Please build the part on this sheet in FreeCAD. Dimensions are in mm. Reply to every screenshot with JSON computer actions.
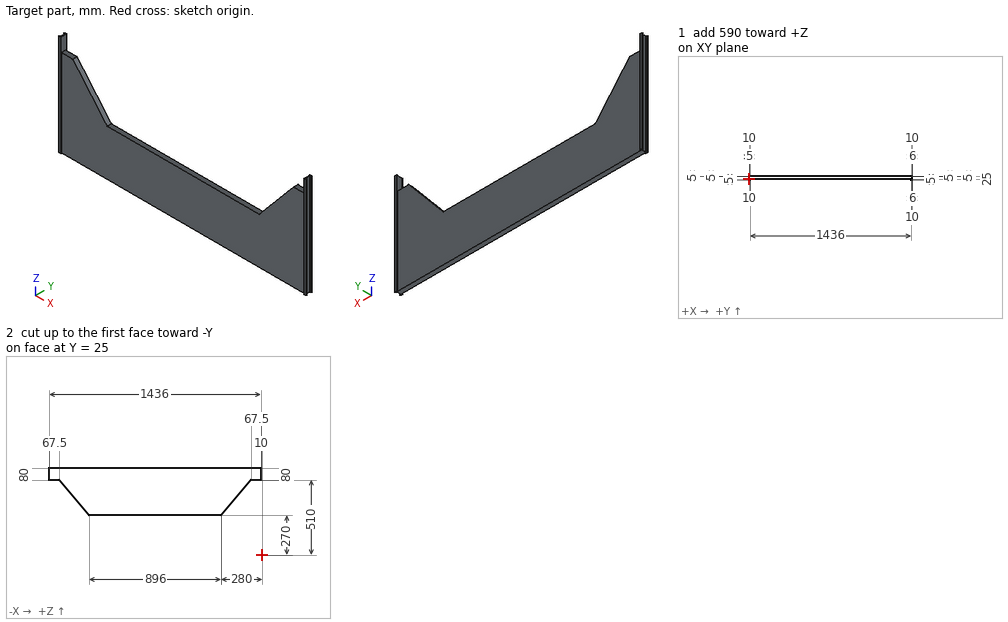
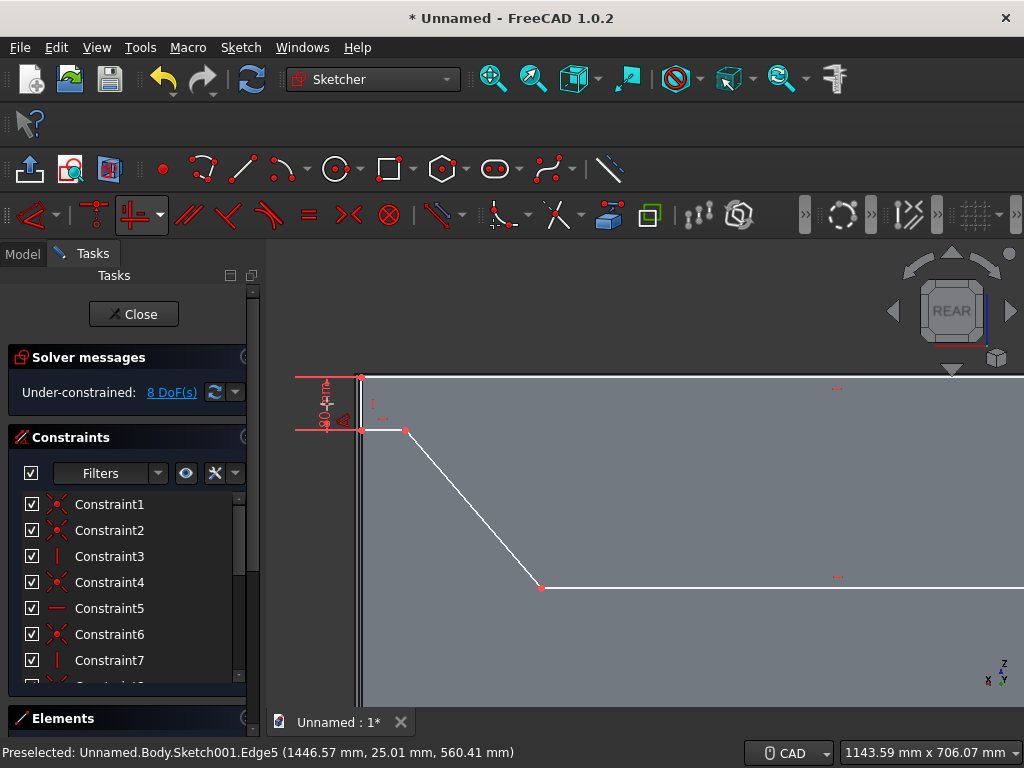
{"action": "left_click", "coordinate": [720, 588]}
{"action": "left_click", "coordinate": [700, 622]}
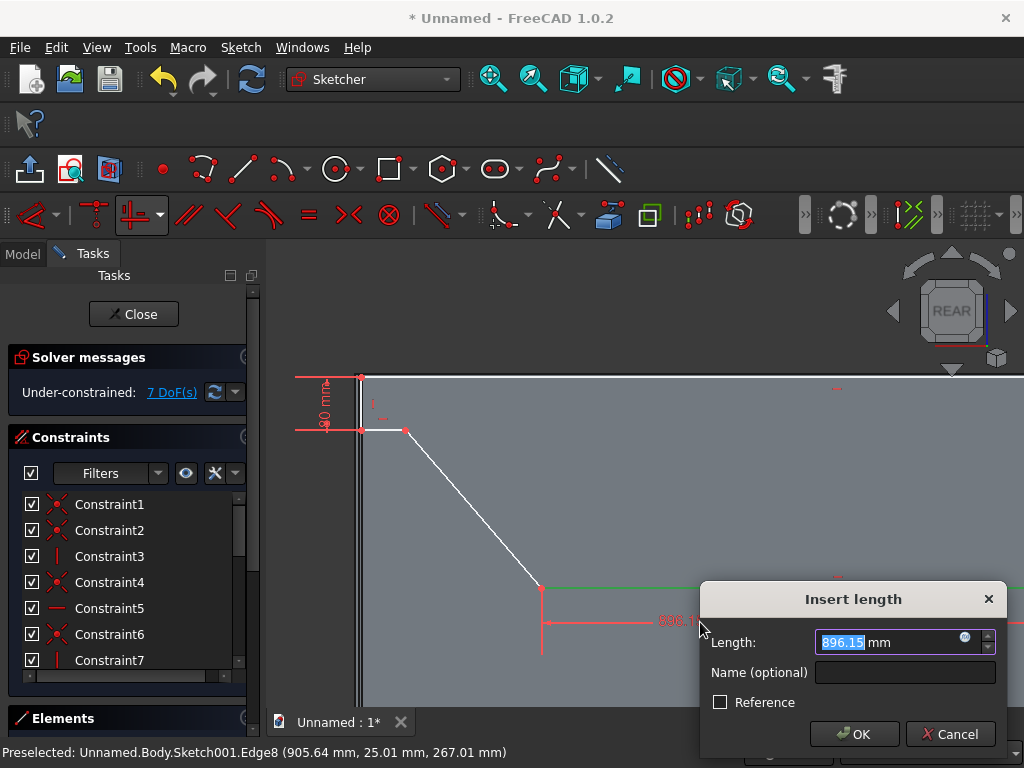
{"action": "type", "text": "896"}
{"action": "key", "text": "Return"}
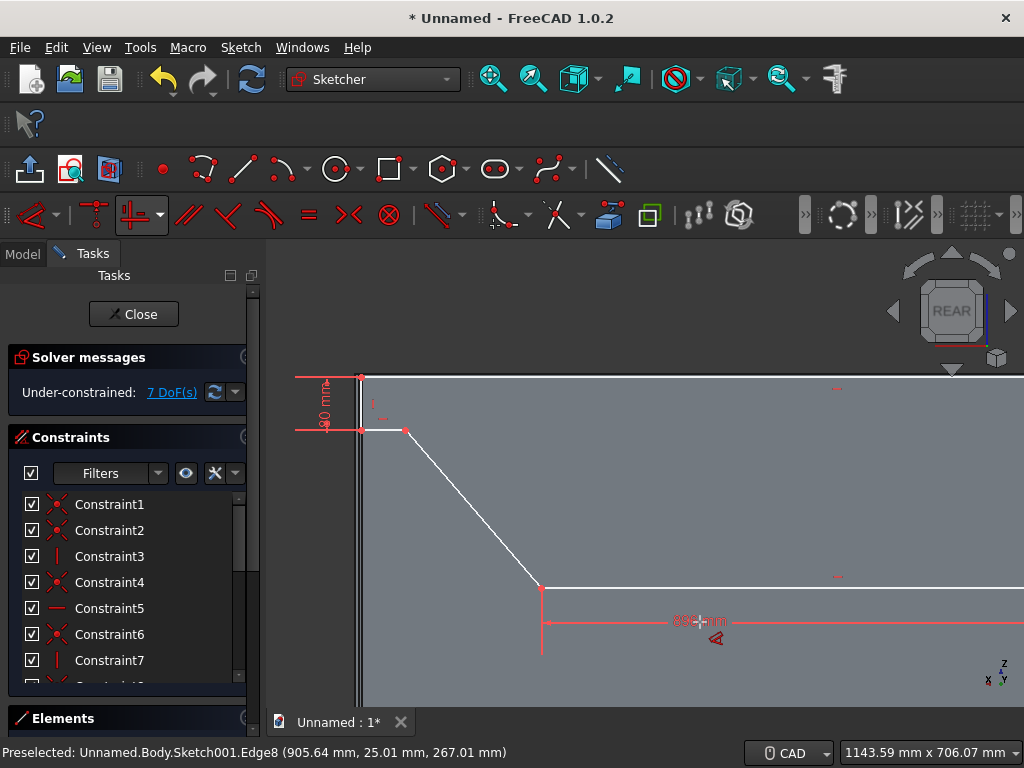
{"action": "scroll", "coordinate": [361, 394], "scroll_direction": "down", "scroll_amount": 4}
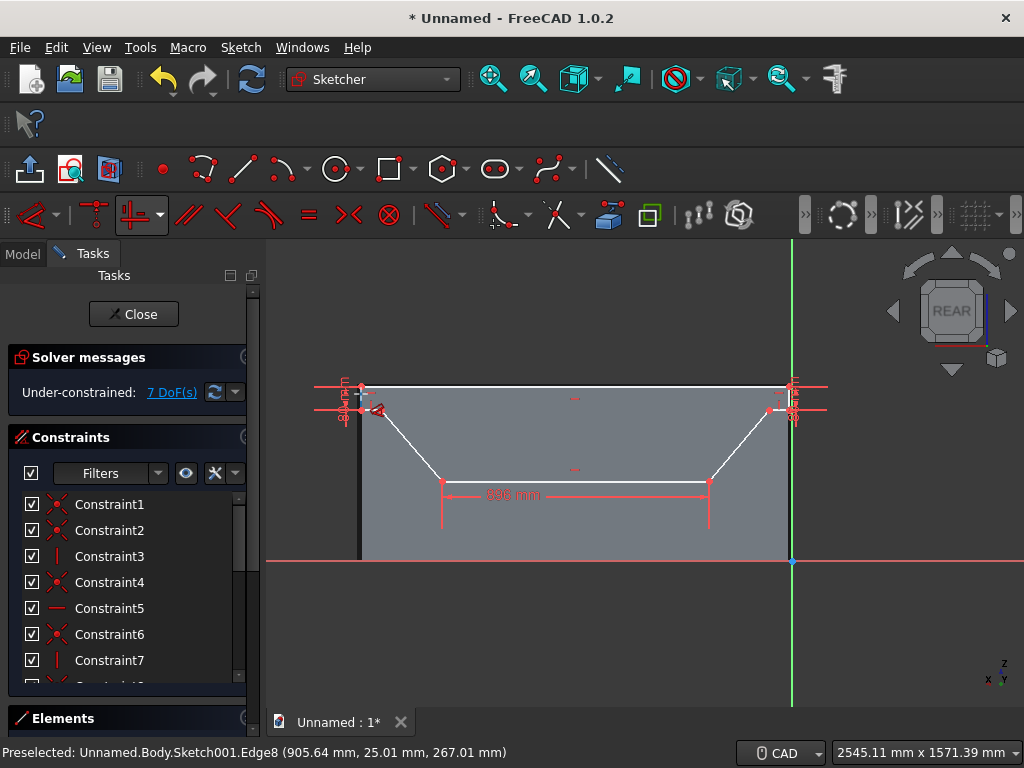
{"action": "scroll", "coordinate": [789, 410], "scroll_direction": "up", "scroll_amount": 13}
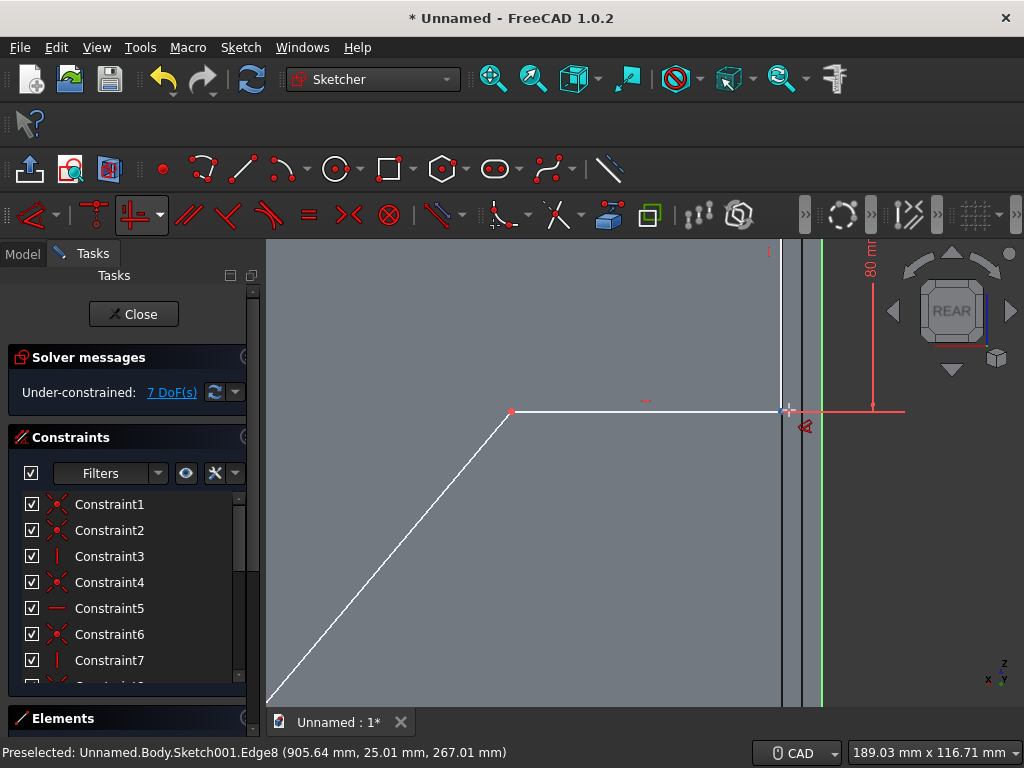
{"action": "left_click", "coordinate": [781, 412]}
{"action": "left_click", "coordinate": [802, 378]}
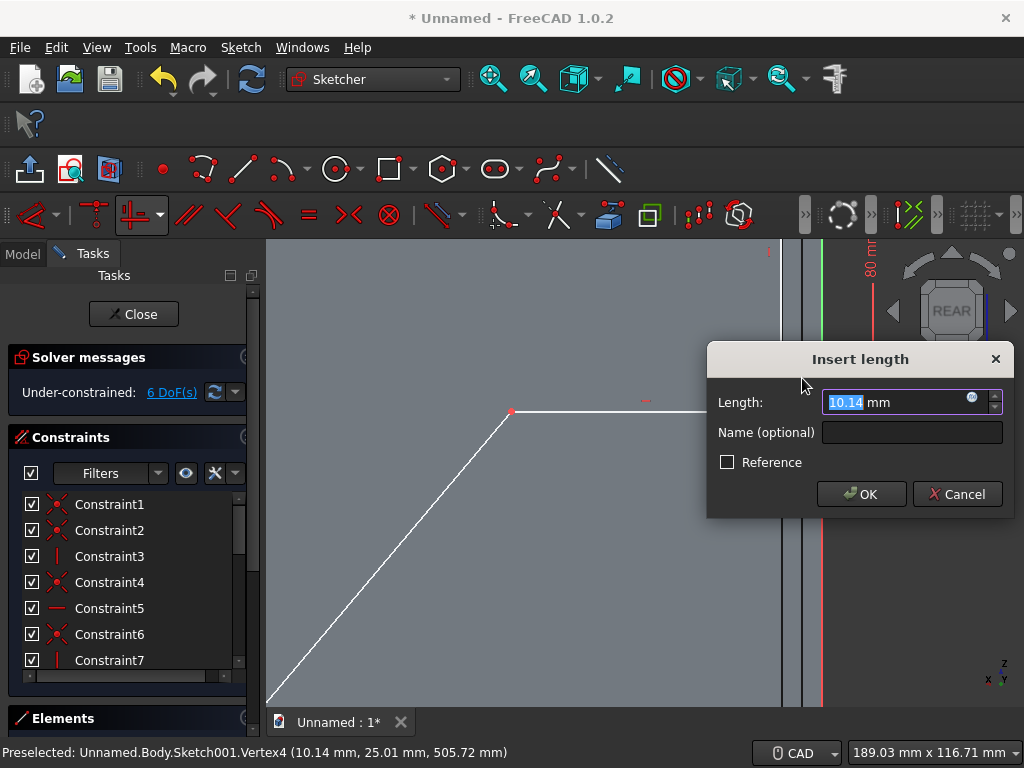
{"action": "type", "text": "10"}
{"action": "key", "text": "Return"}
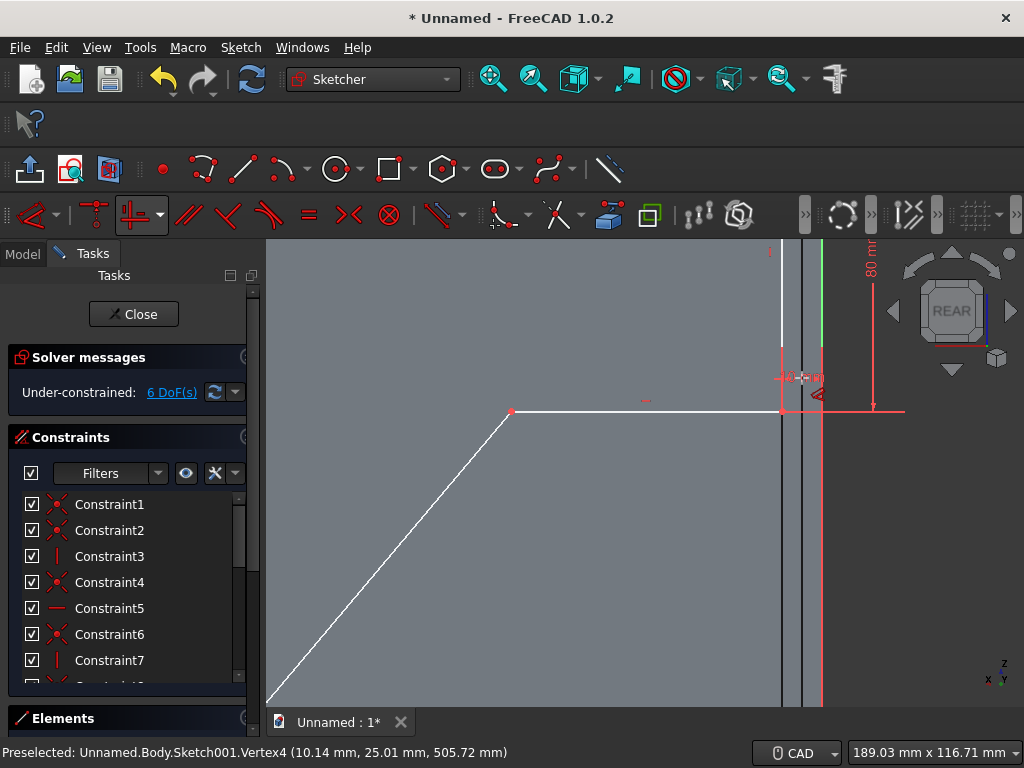
{"action": "scroll", "coordinate": [789, 410], "scroll_direction": "down", "scroll_amount": 13}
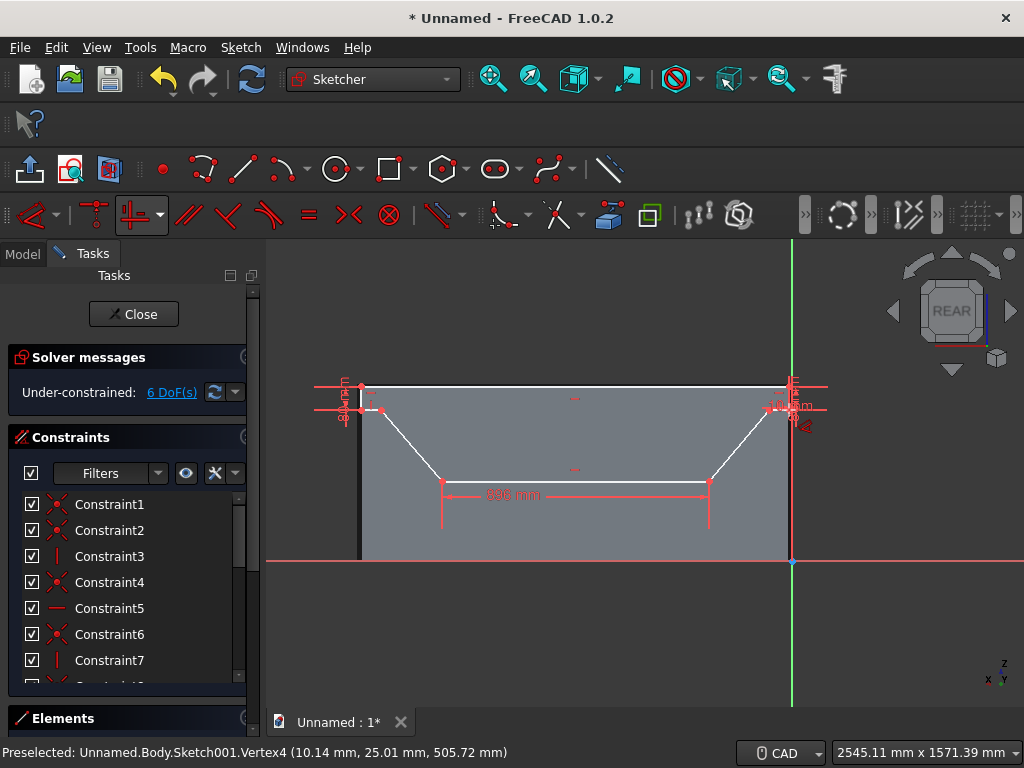
{"action": "scroll", "coordinate": [775, 410], "scroll_direction": "up", "scroll_amount": 5}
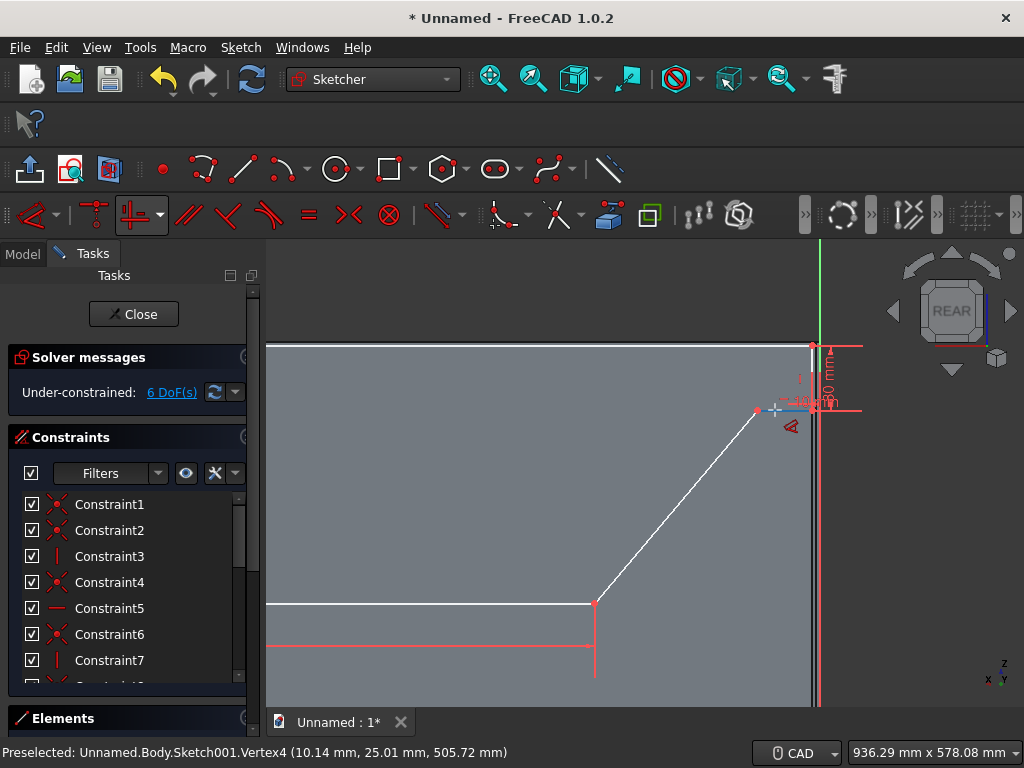
{"action": "left_click", "coordinate": [774, 411]}
{"action": "left_click", "coordinate": [785, 445]}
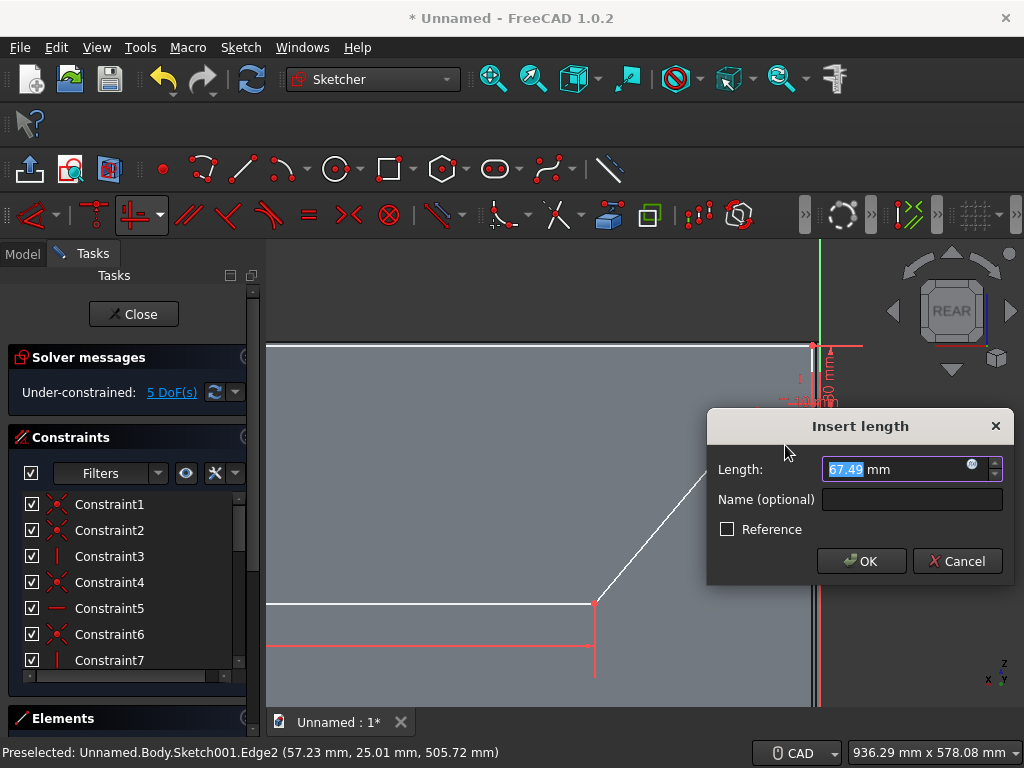
{"action": "type", "text": "67.5"}
{"action": "key", "text": "Return"}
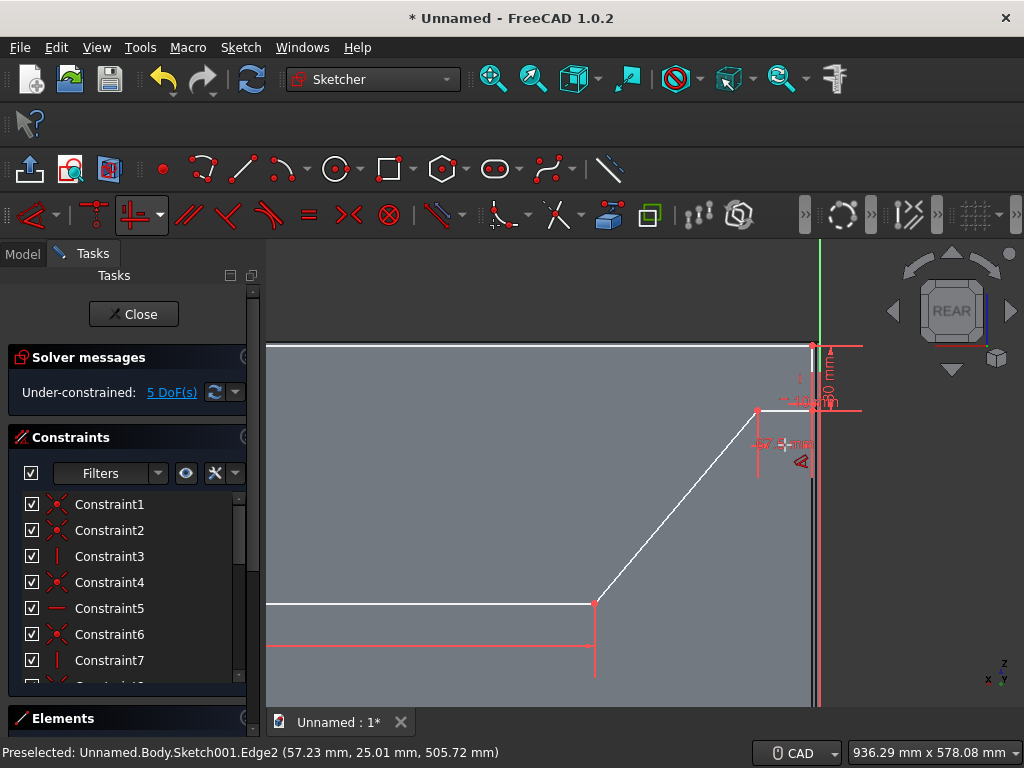
{"action": "left_click", "coordinate": [463, 346]}
{"action": "left_click", "coordinate": [553, 312]}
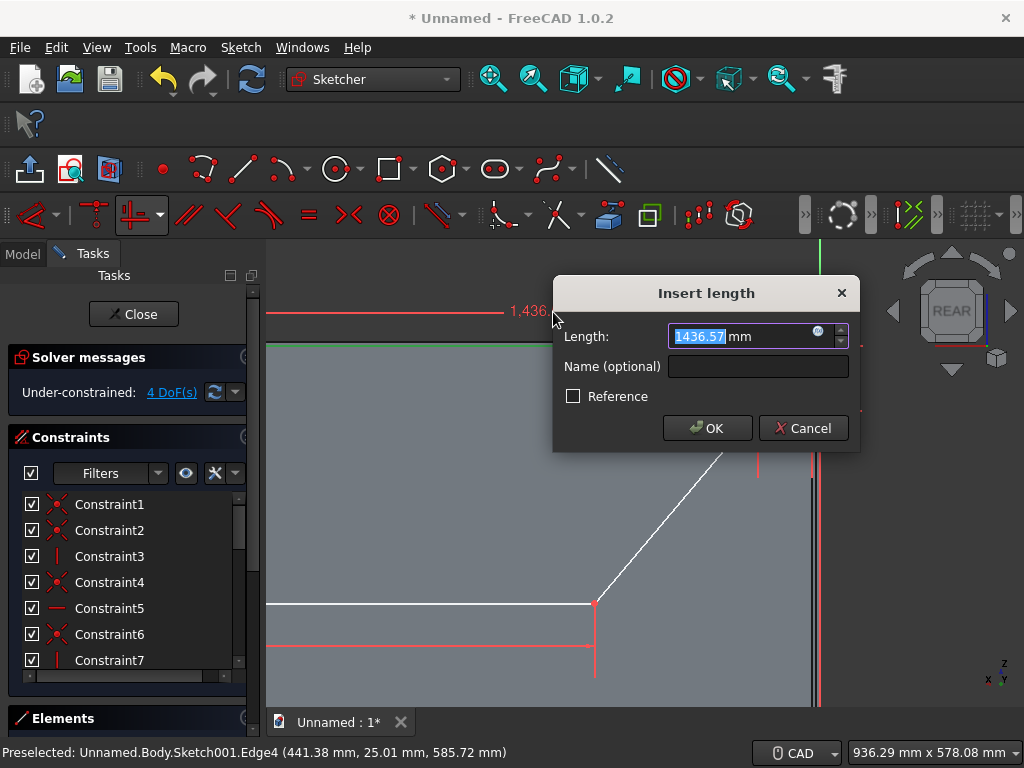
{"action": "type", "text": "1436"}
{"action": "key", "text": "Return"}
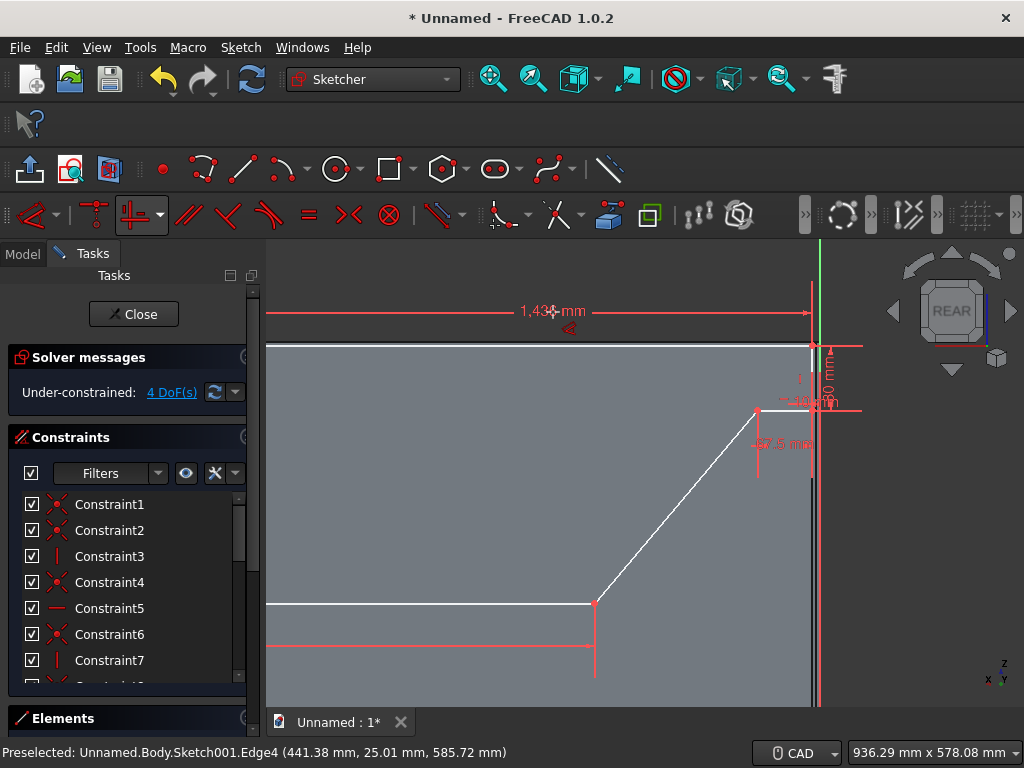
{"action": "scroll", "coordinate": [775, 410], "scroll_direction": "down", "scroll_amount": 5}